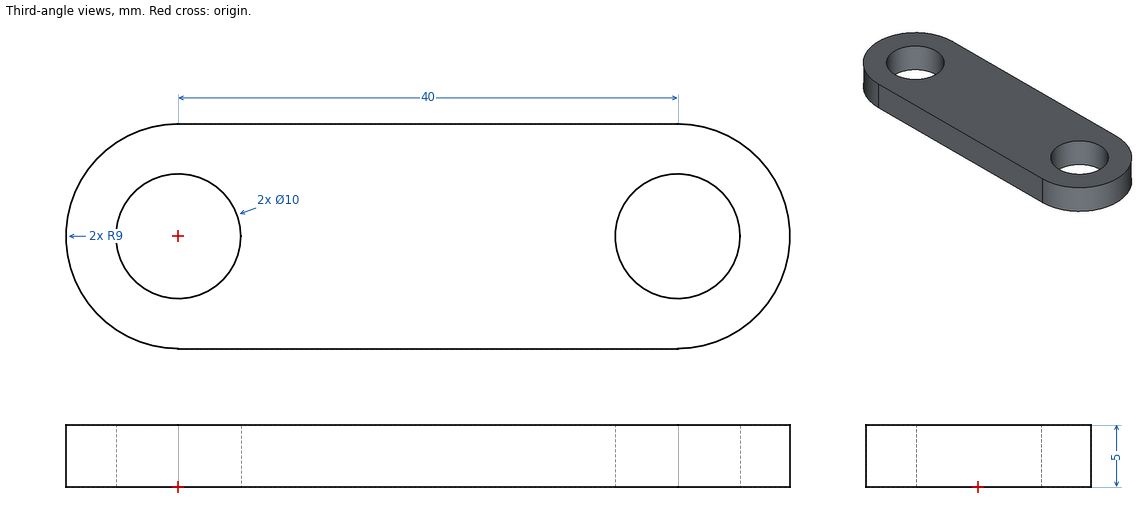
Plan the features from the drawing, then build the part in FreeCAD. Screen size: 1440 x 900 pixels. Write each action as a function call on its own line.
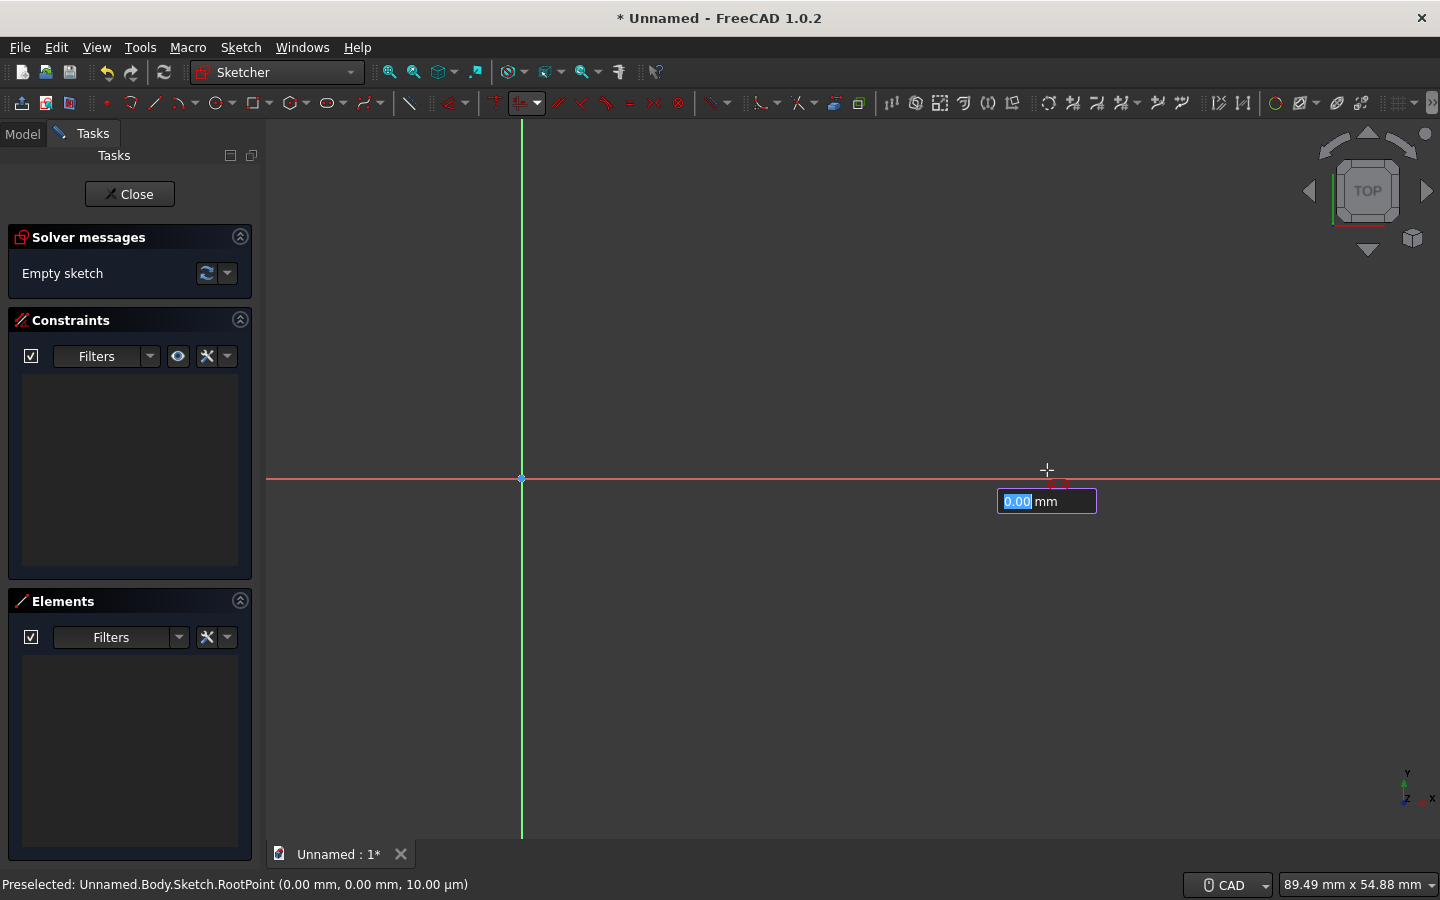
click(784, 361)
key(Escape)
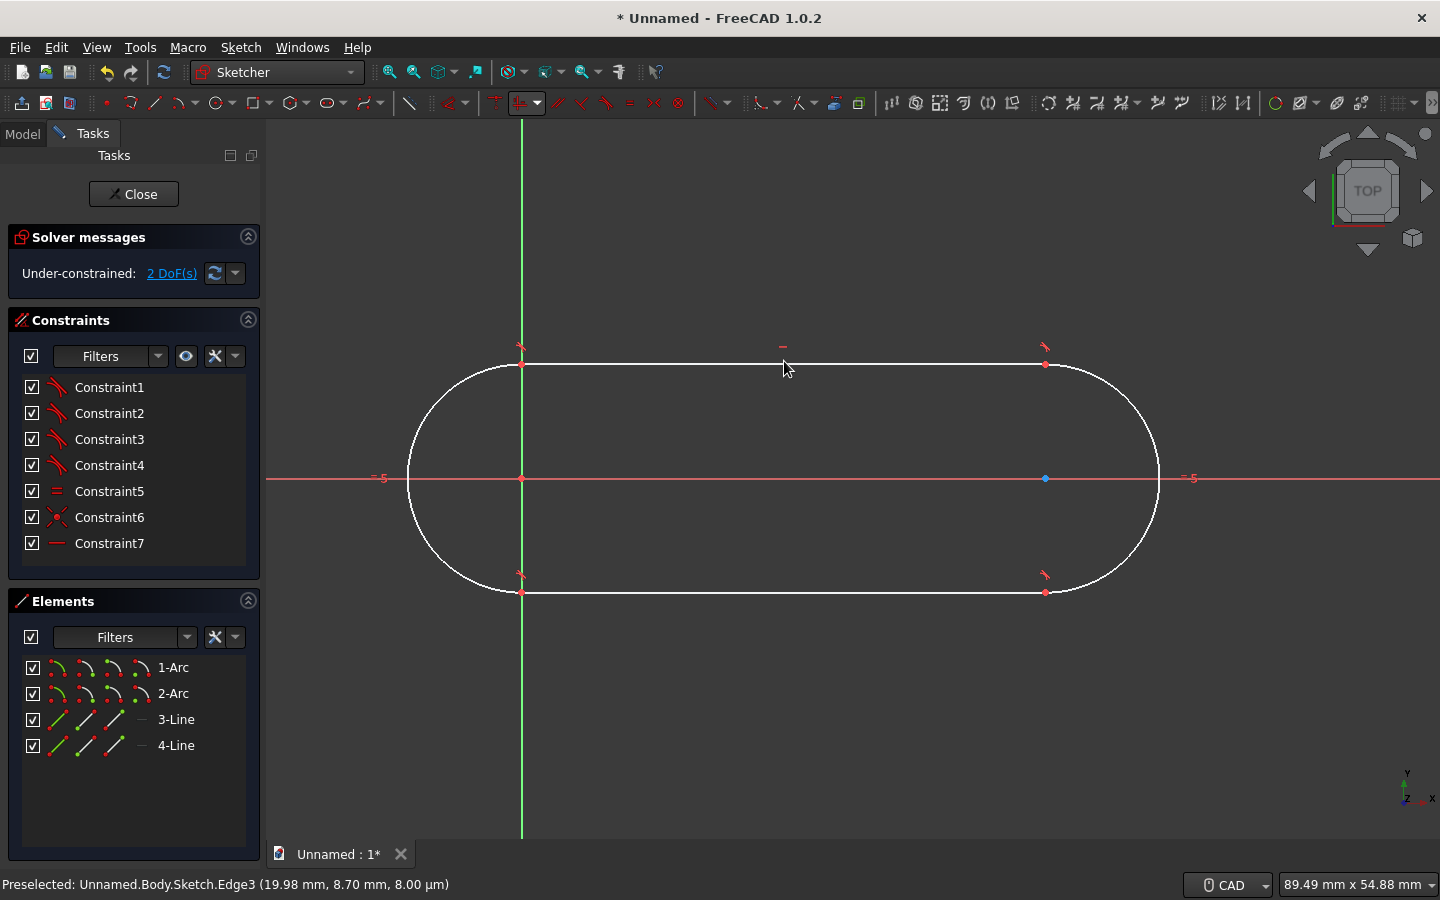
click(448, 104)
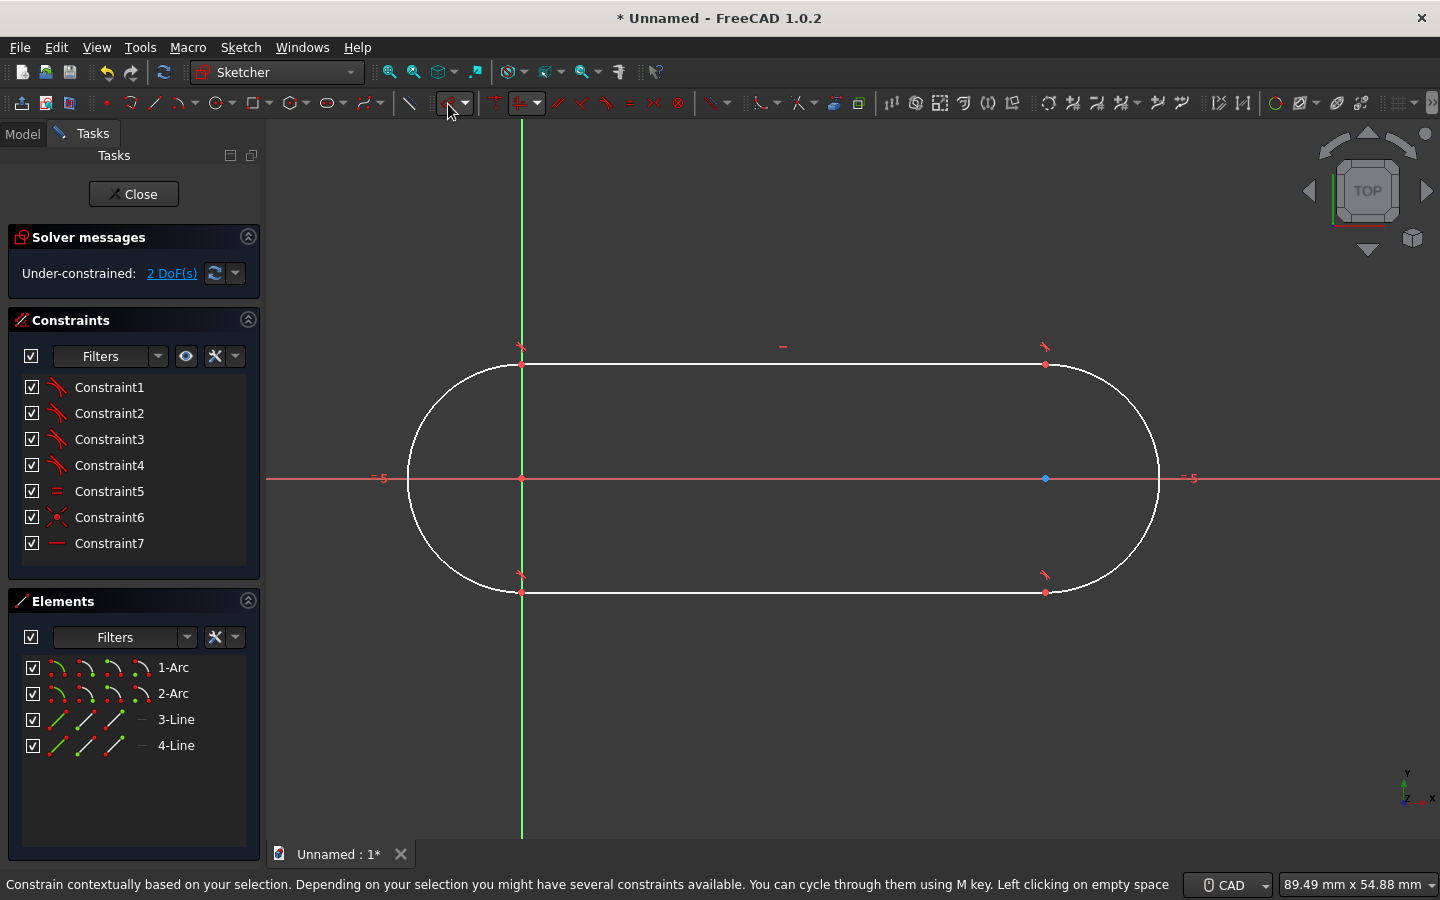
click(429, 412)
click(403, 393)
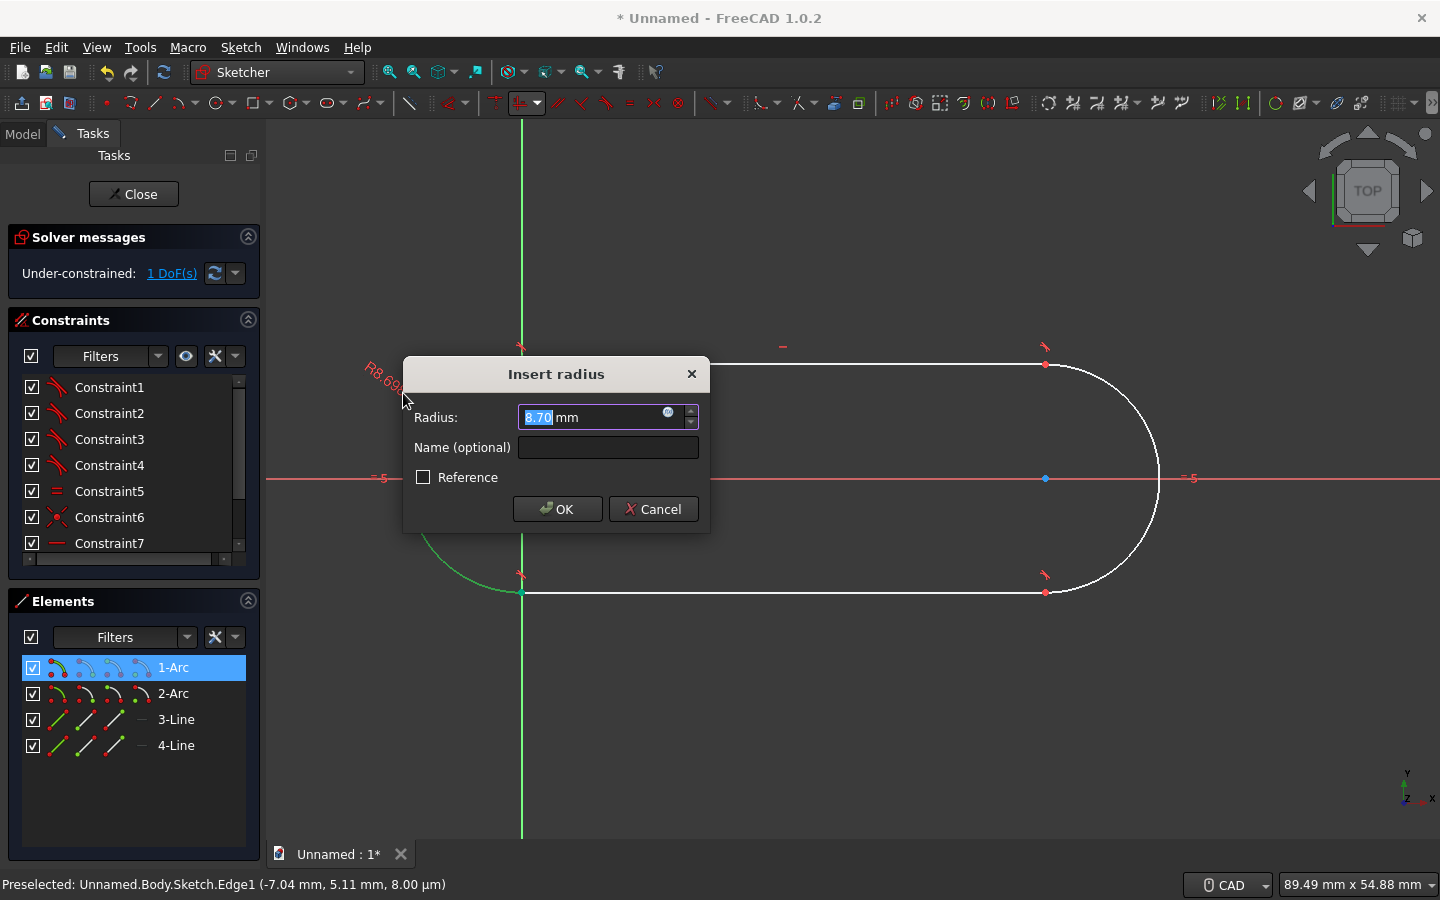
text(9)
key(Return)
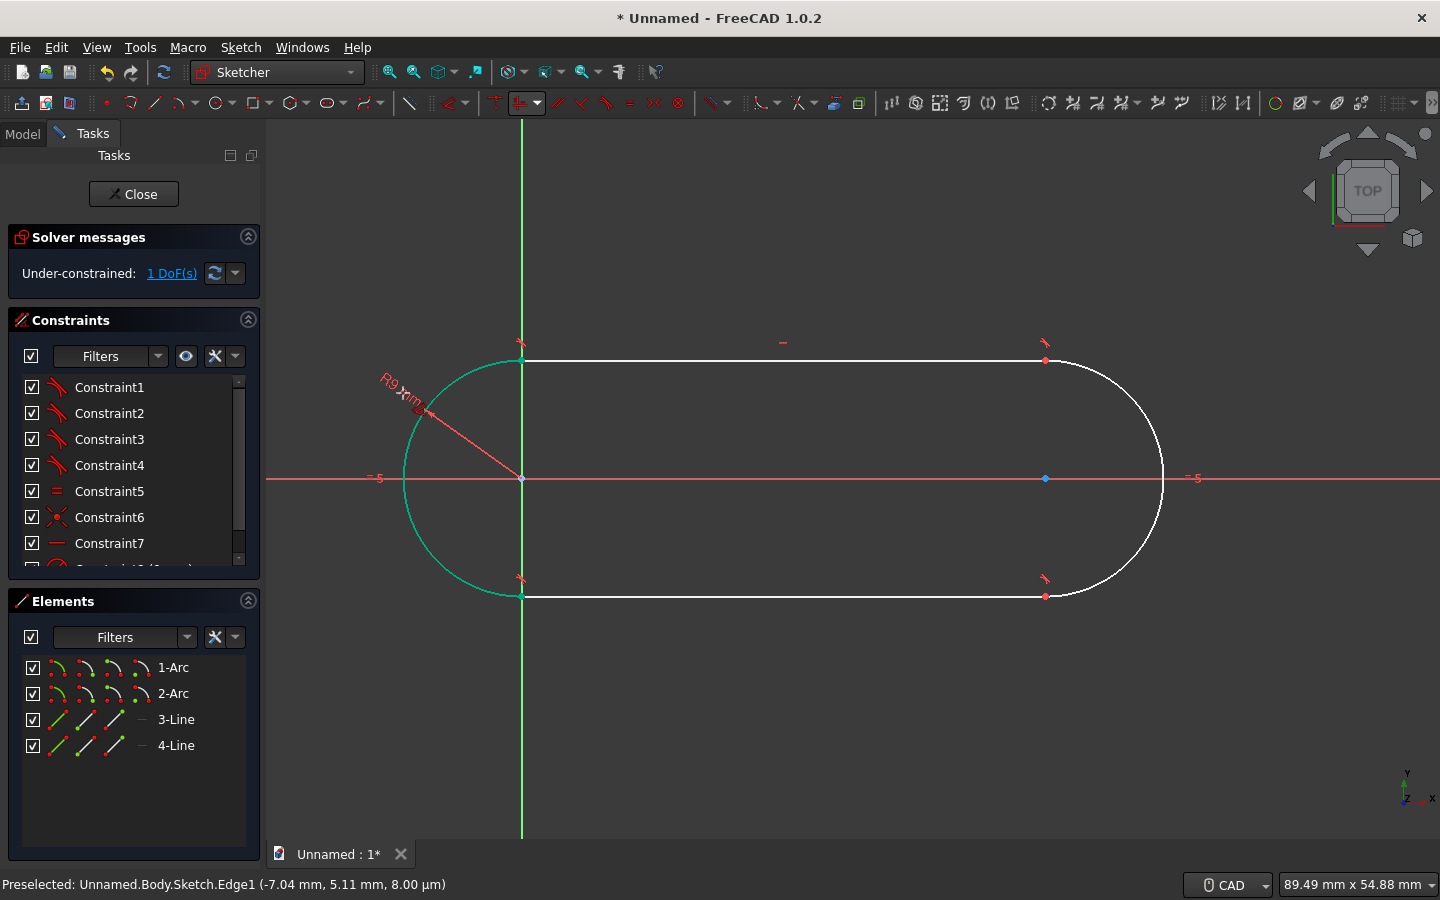
click(679, 361)
click(784, 327)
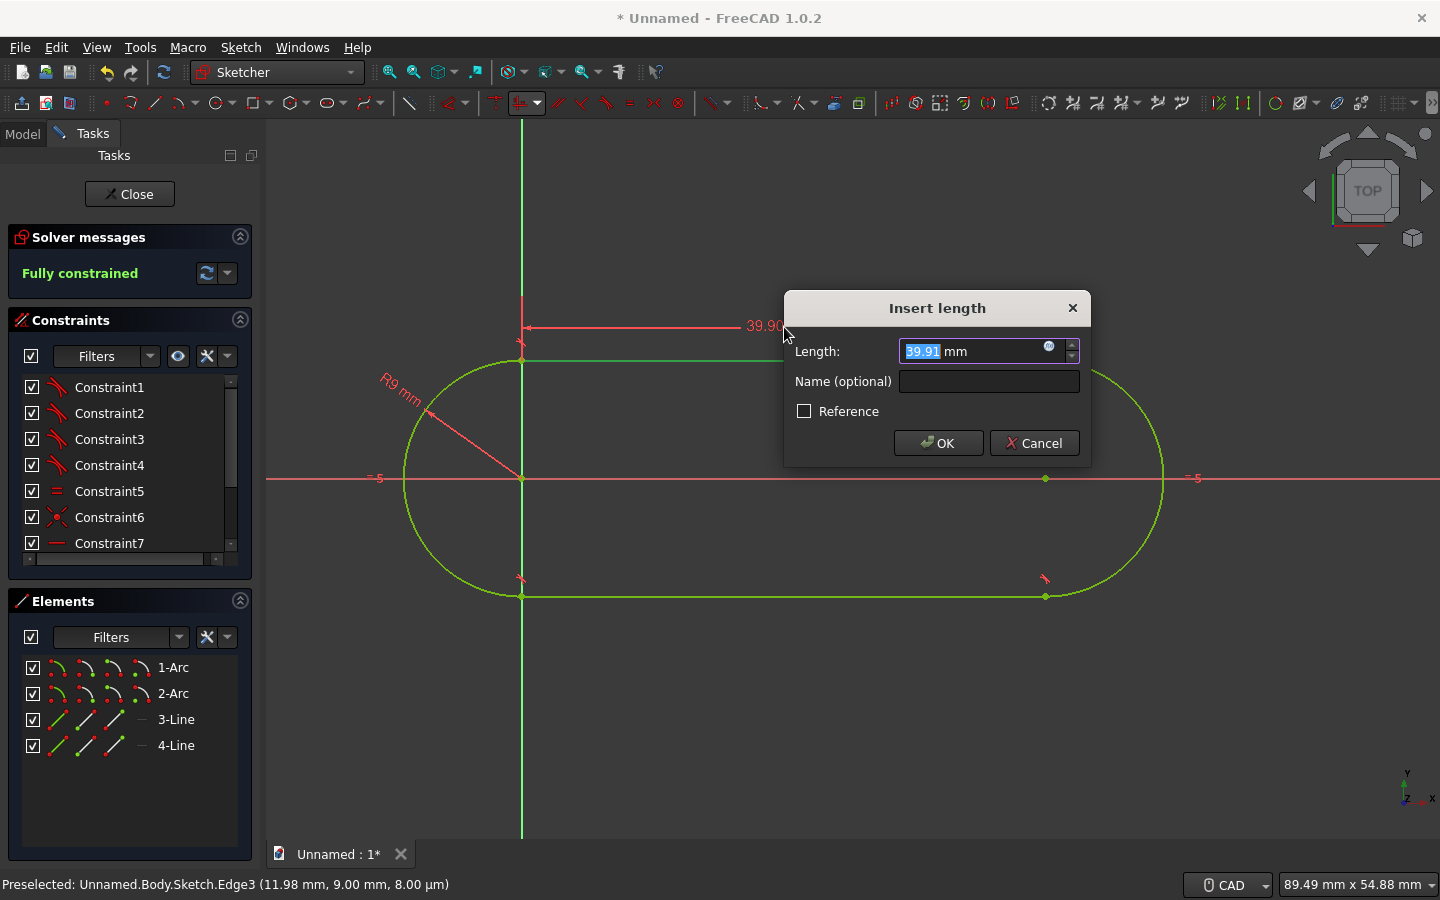
text(40)
key(Return)
key(Escape)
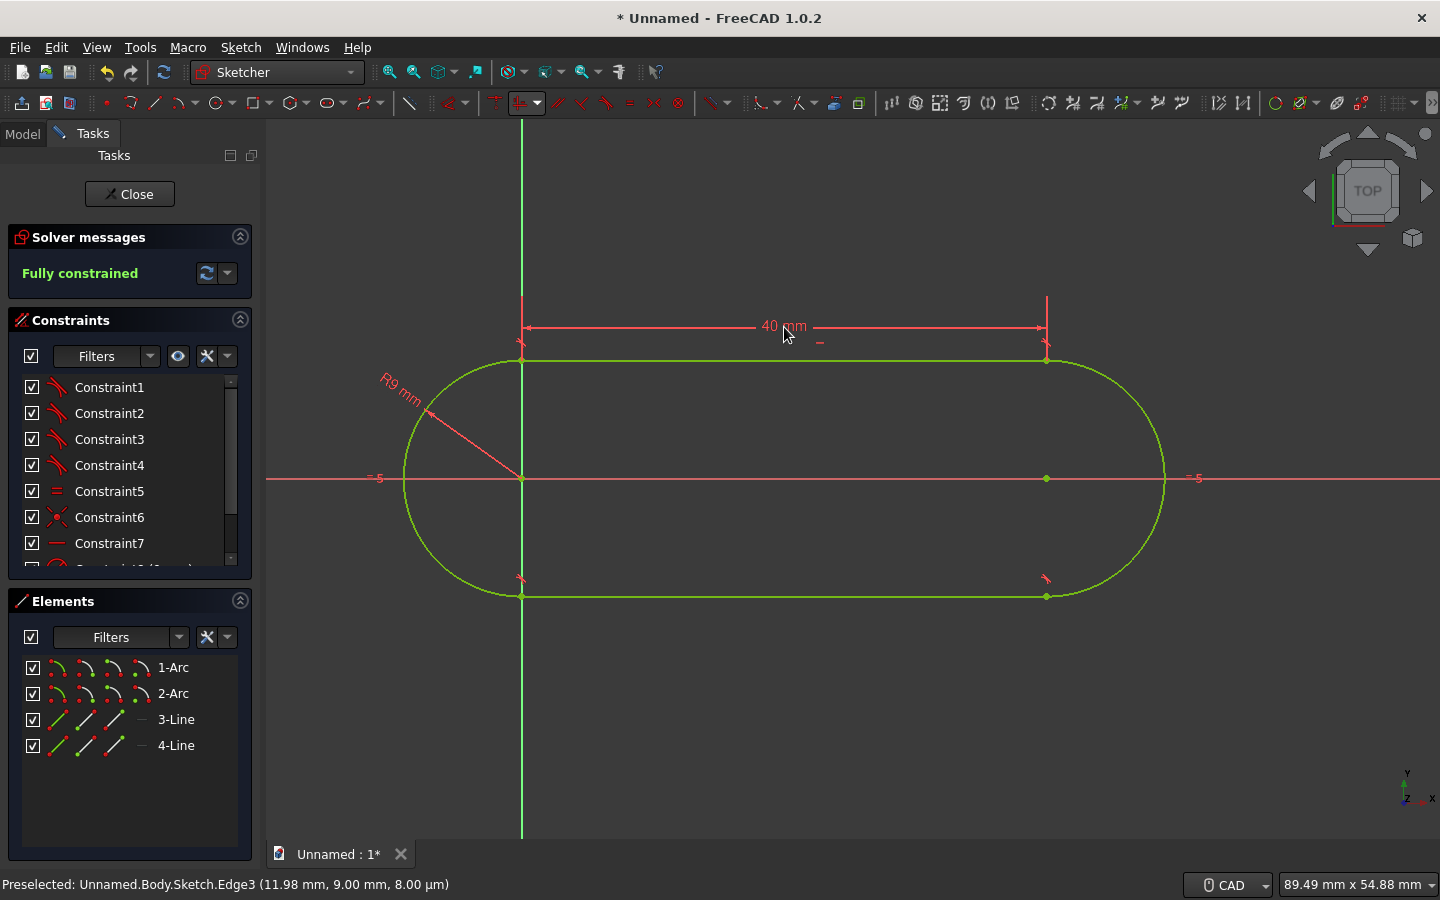
click(130, 194)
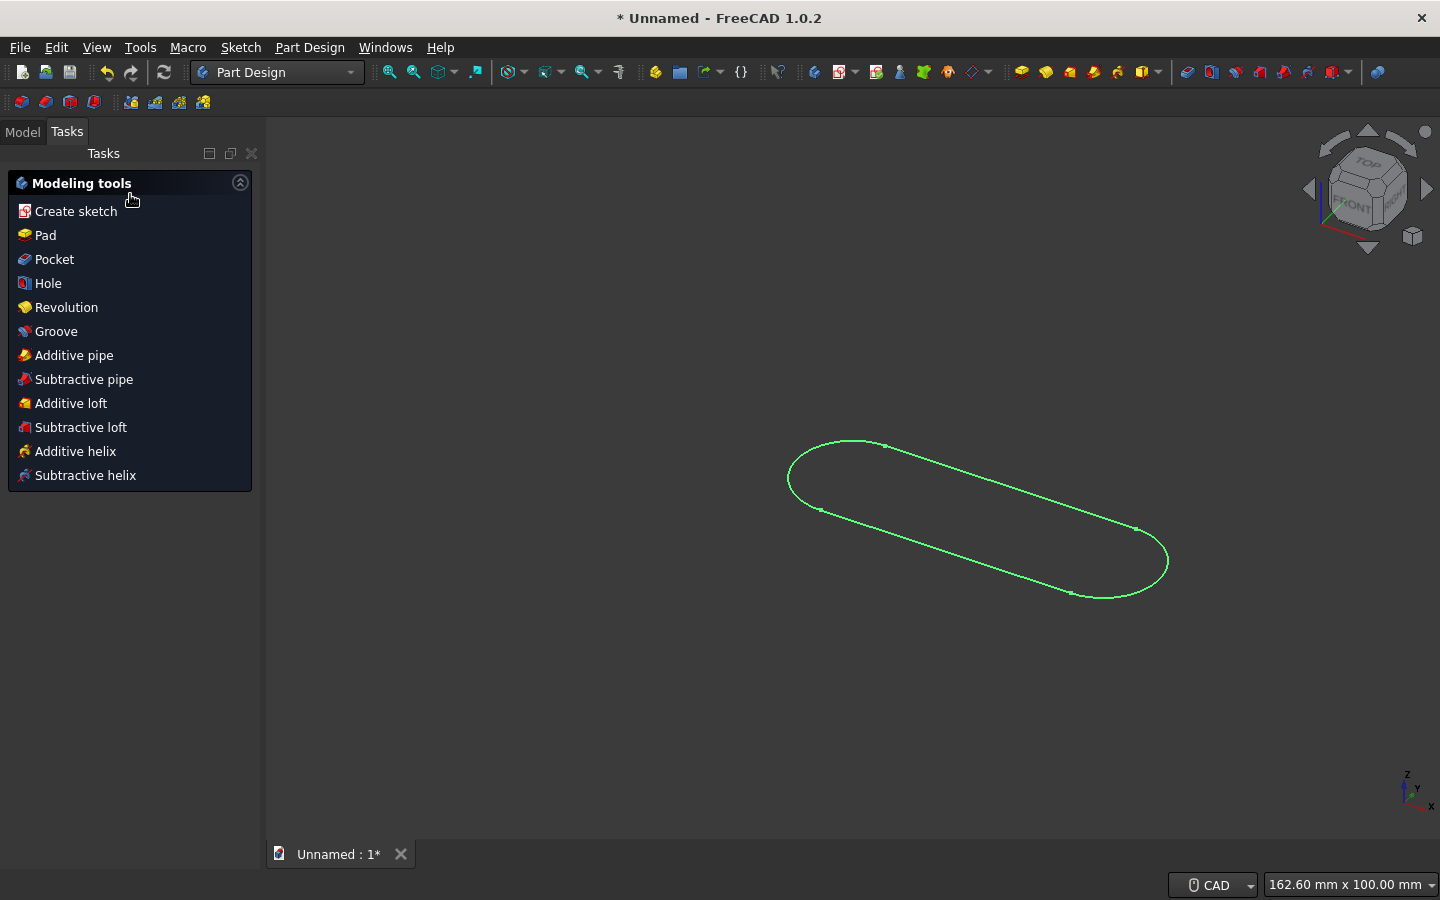
click(1022, 72)